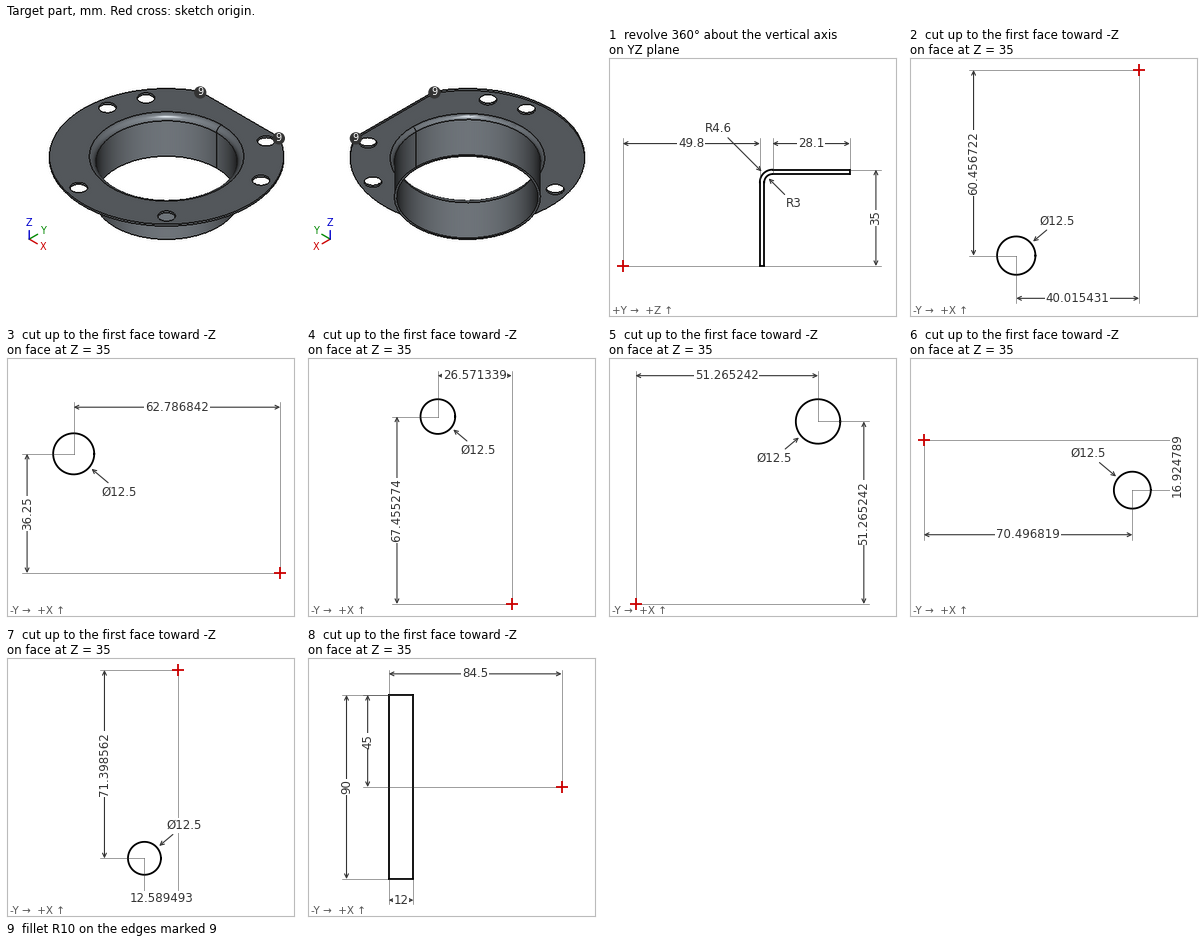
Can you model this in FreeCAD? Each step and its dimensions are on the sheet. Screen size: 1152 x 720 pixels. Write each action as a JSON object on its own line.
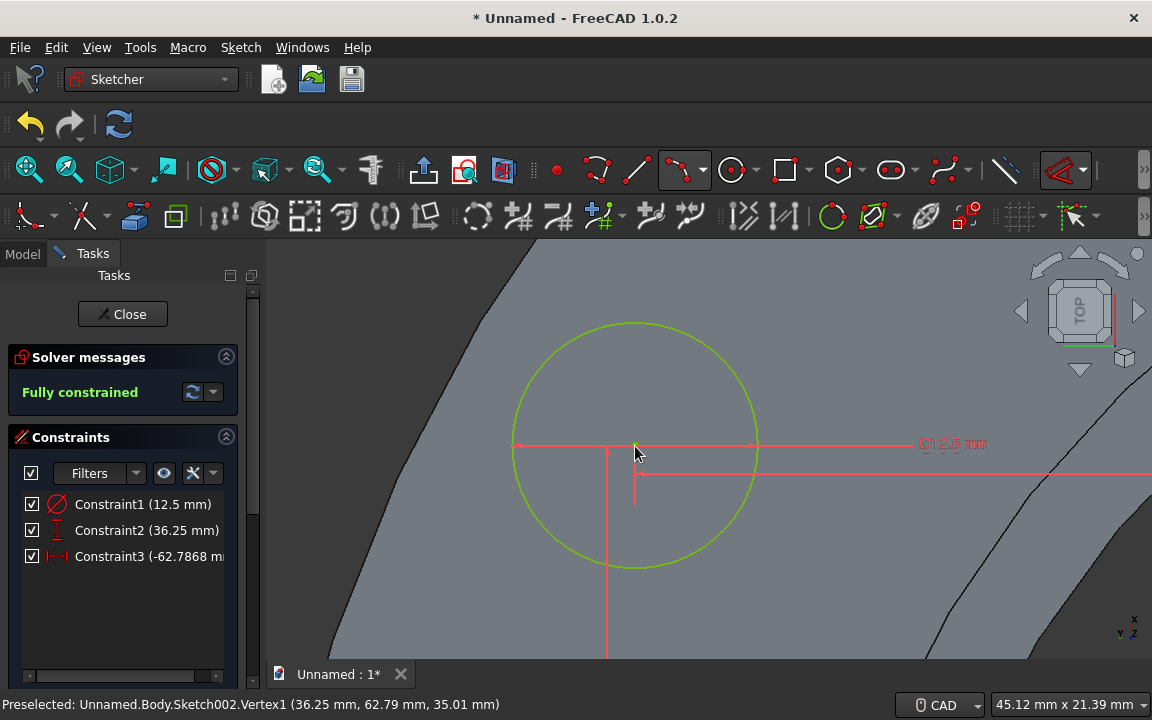
{"action": "left_click", "coordinate": [123, 314]}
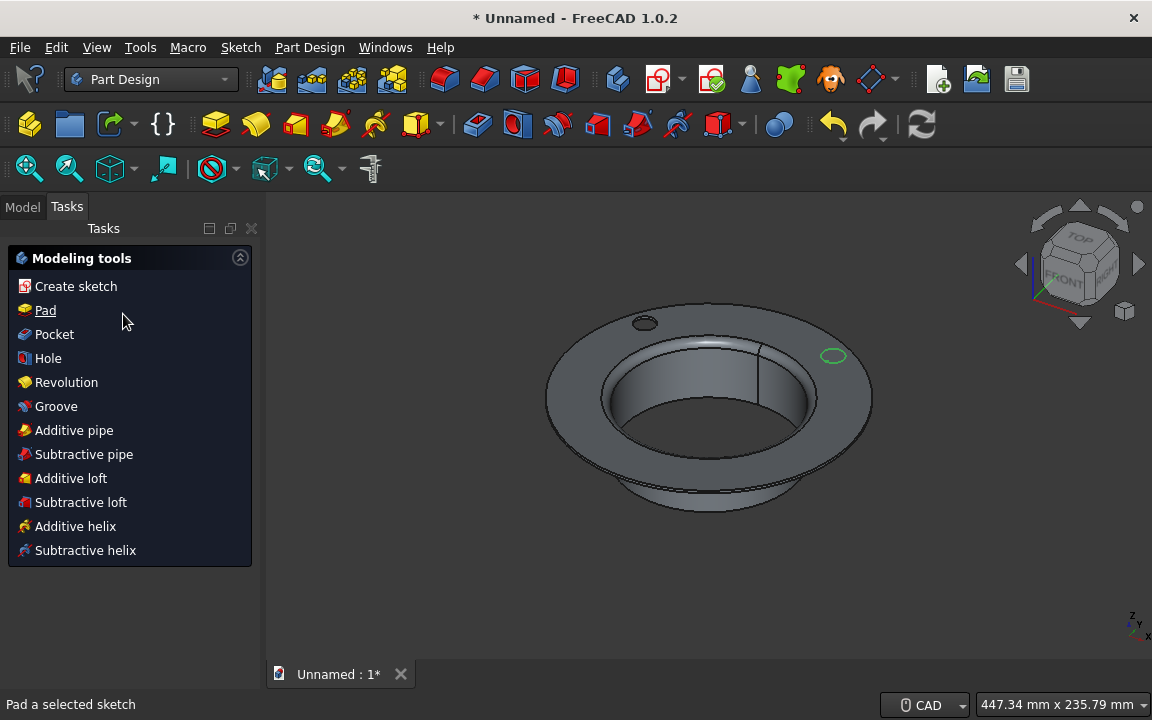
{"action": "left_click", "coordinate": [478, 124]}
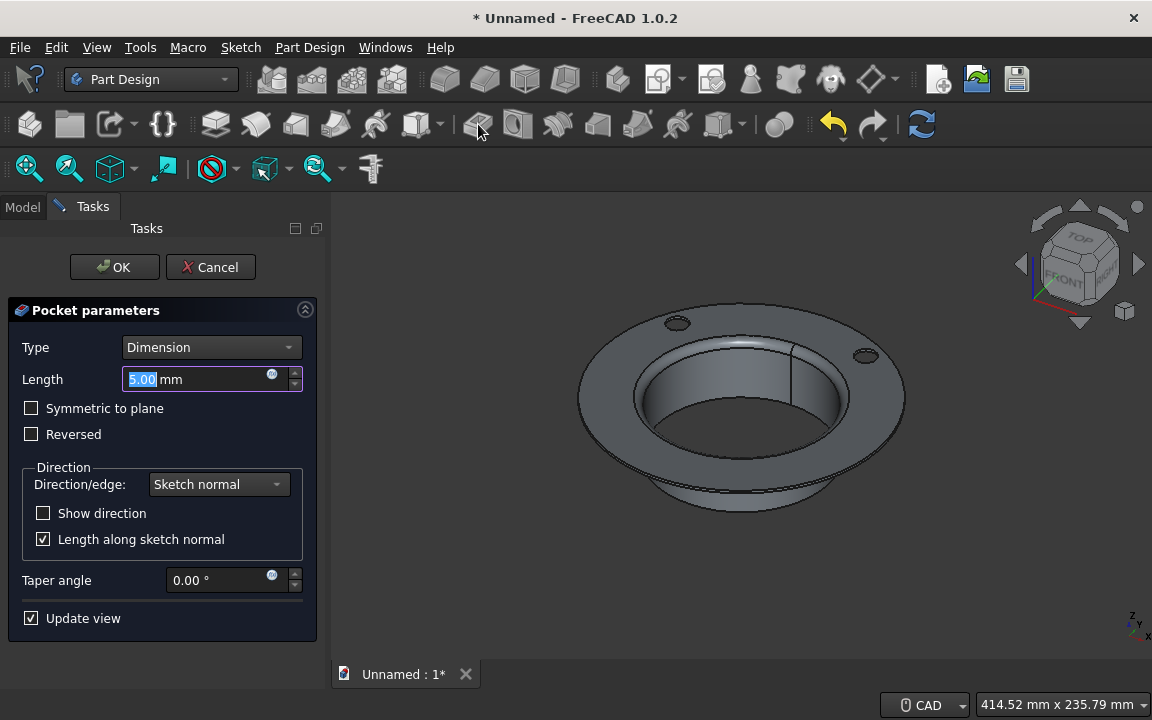
{"action": "left_click", "coordinate": [212, 348]}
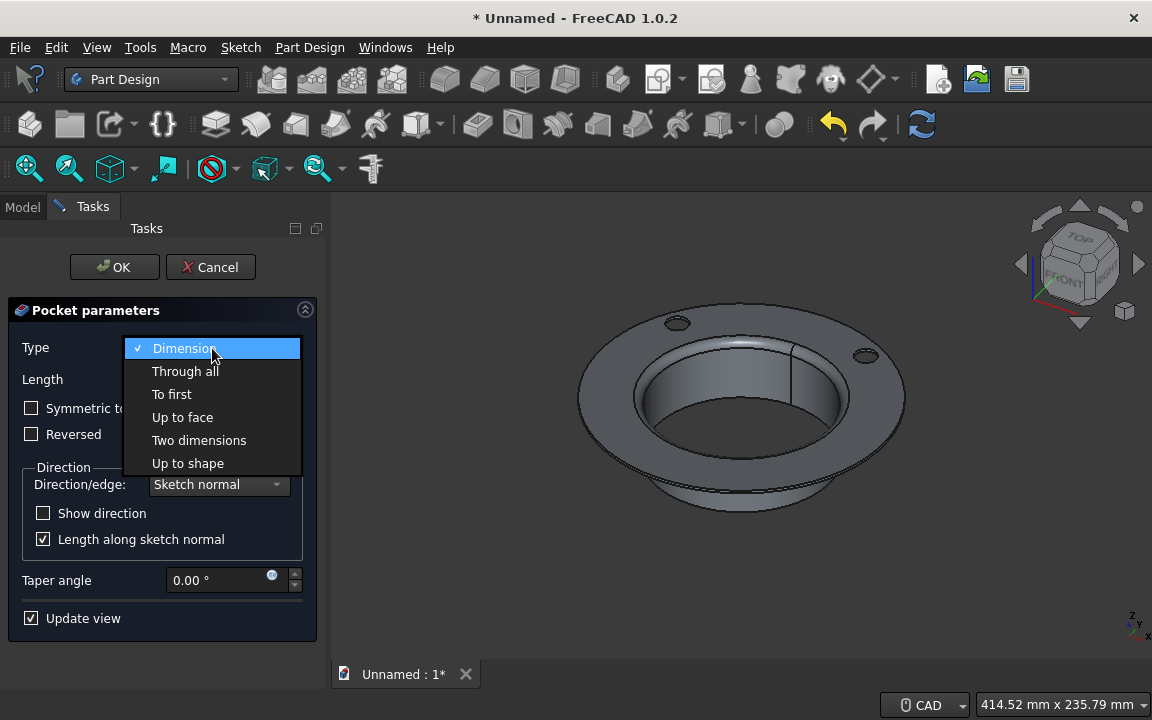
{"action": "left_click", "coordinate": [212, 394]}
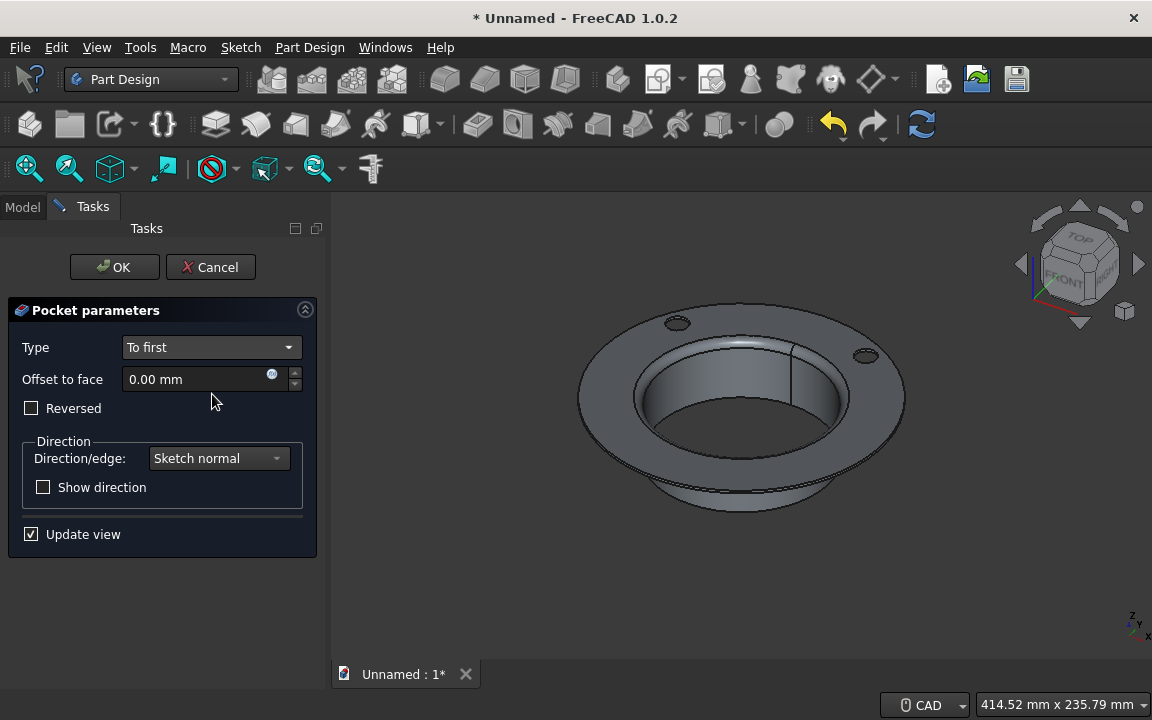
{"action": "left_click", "coordinate": [115, 267]}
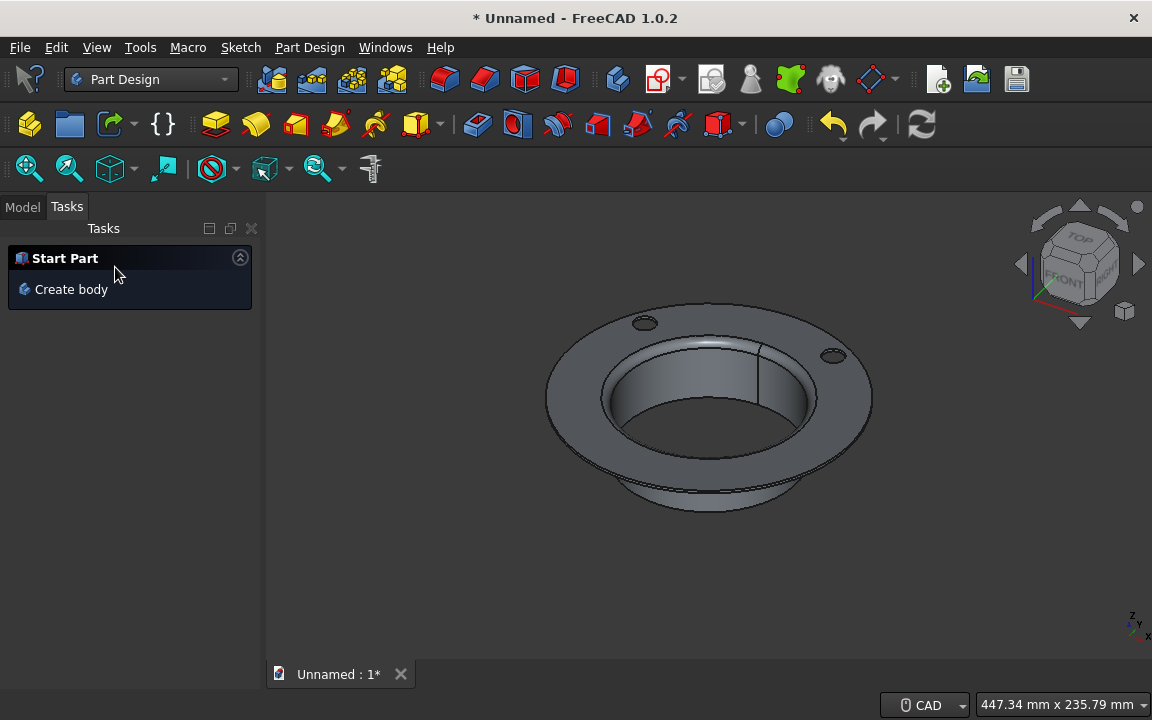
{"action": "left_click", "coordinate": [743, 469]}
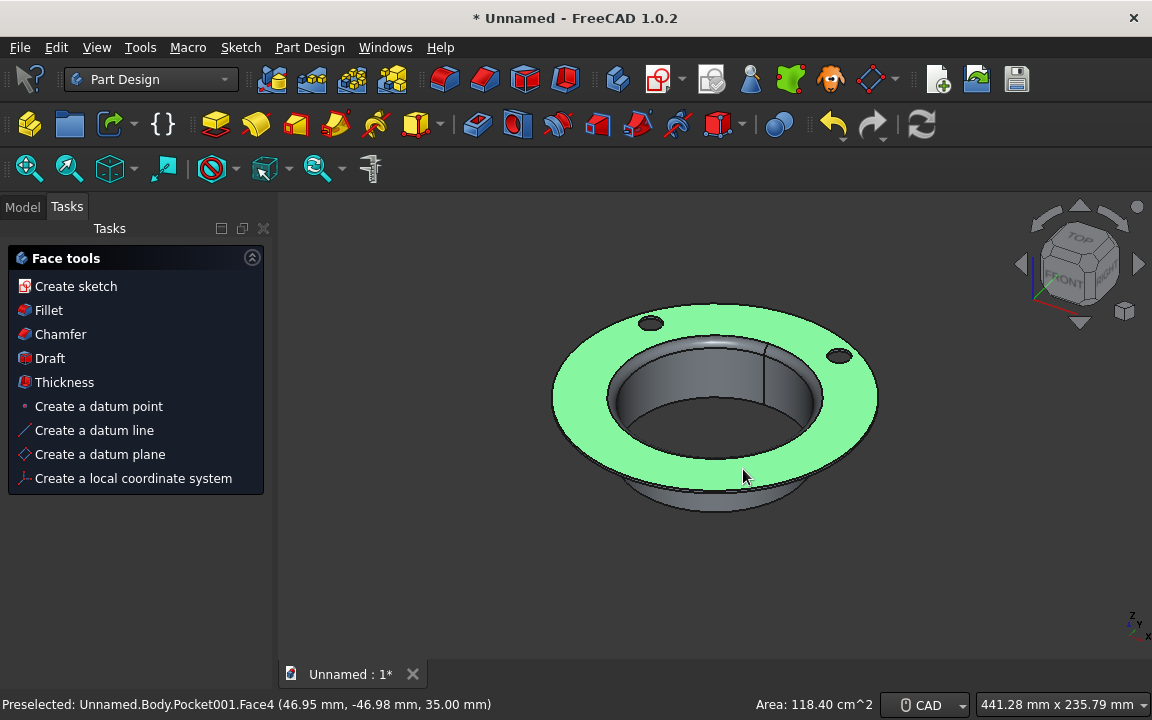
{"action": "left_click", "coordinate": [658, 80]}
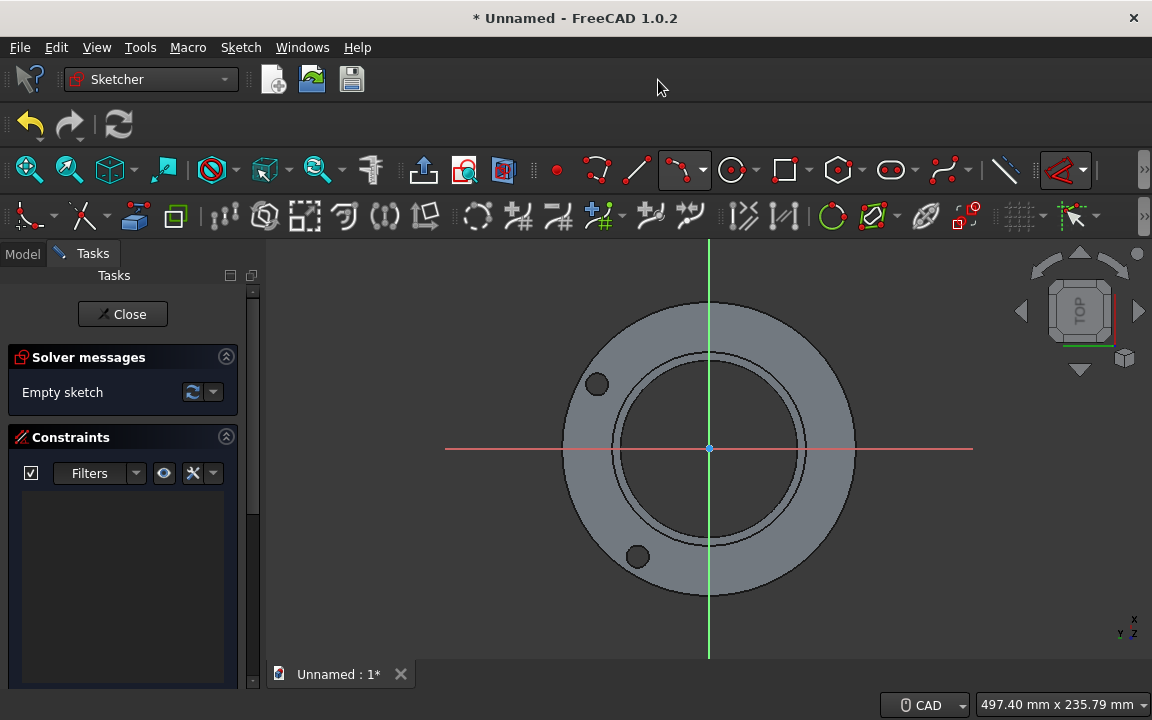
{"action": "scroll", "coordinate": [664, 317], "scroll_direction": "up", "scroll_amount": 12}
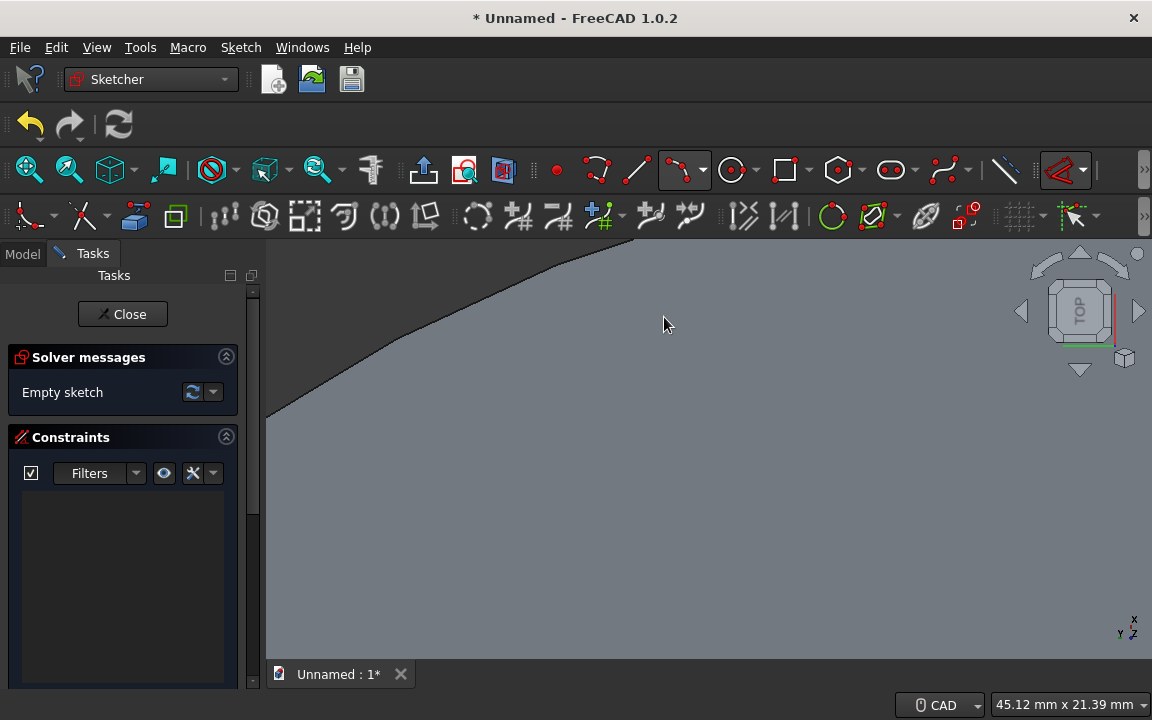
{"action": "left_click", "coordinate": [732, 170]}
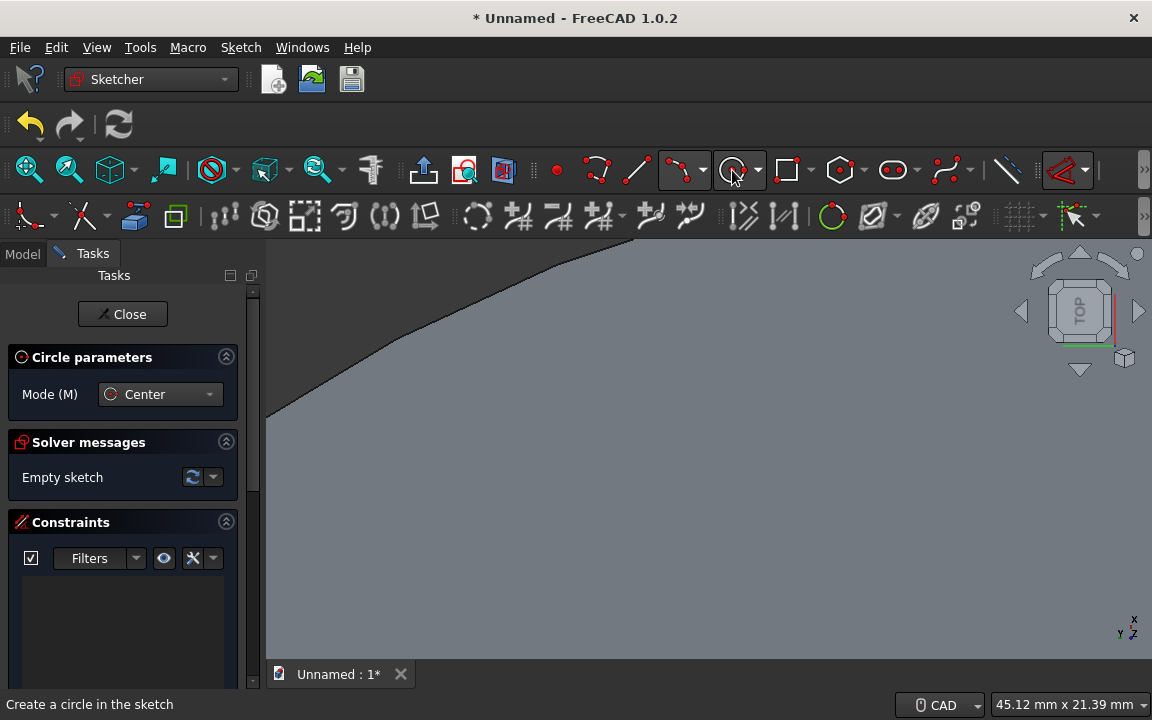
{"action": "left_click", "coordinate": [634, 446]}
{"action": "mouse_move", "coordinate": [721, 359]}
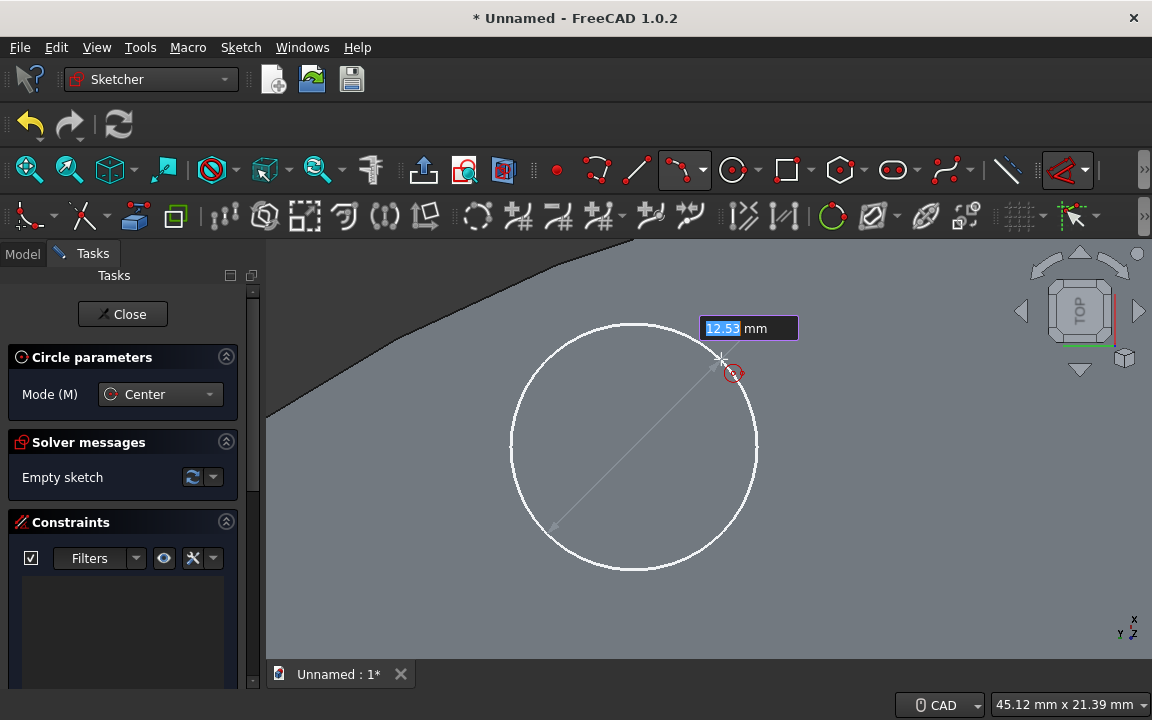
{"action": "type", "text": "12.5"}
{"action": "key", "text": "Return"}
{"action": "key", "text": "Escape"}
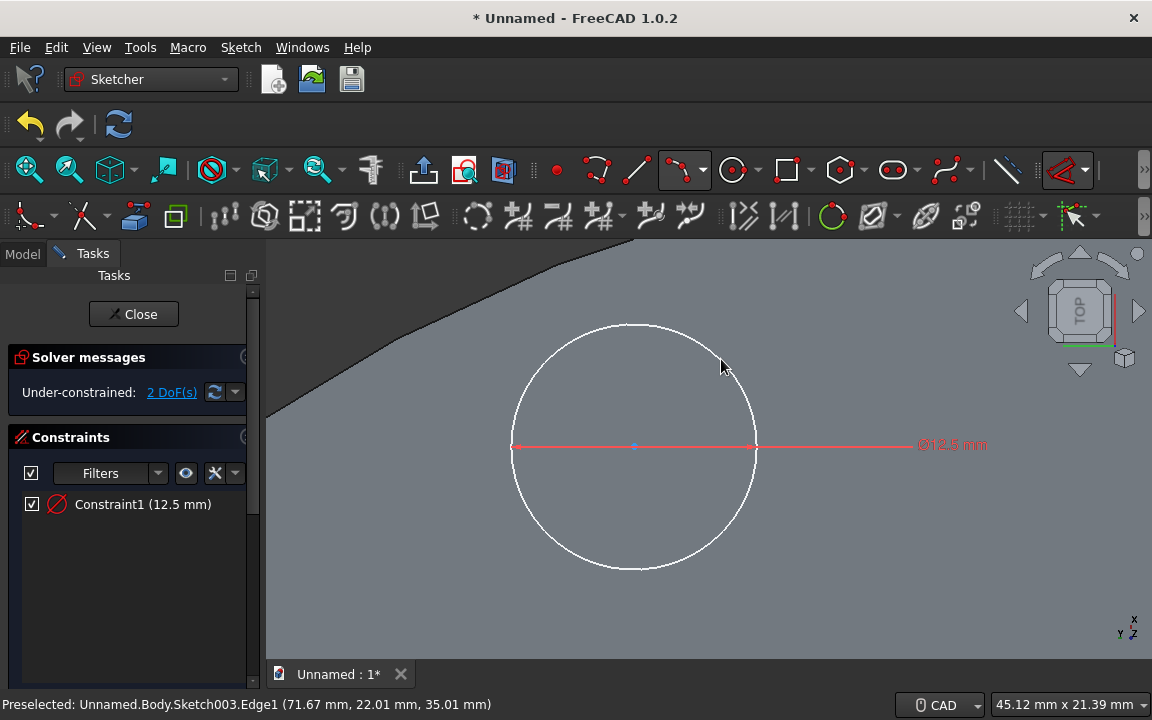
{"action": "left_click", "coordinate": [634, 447]}